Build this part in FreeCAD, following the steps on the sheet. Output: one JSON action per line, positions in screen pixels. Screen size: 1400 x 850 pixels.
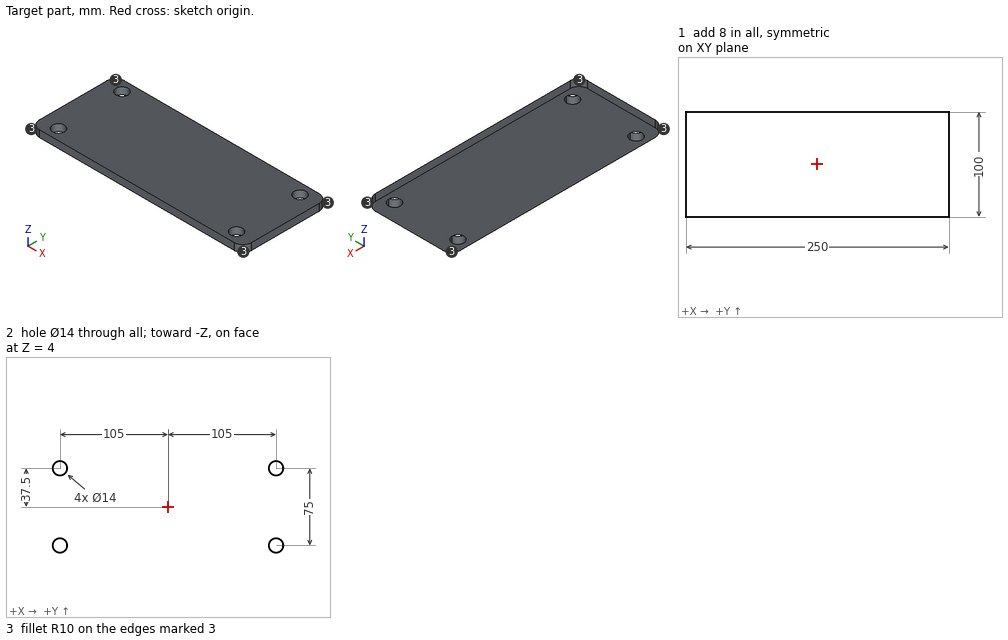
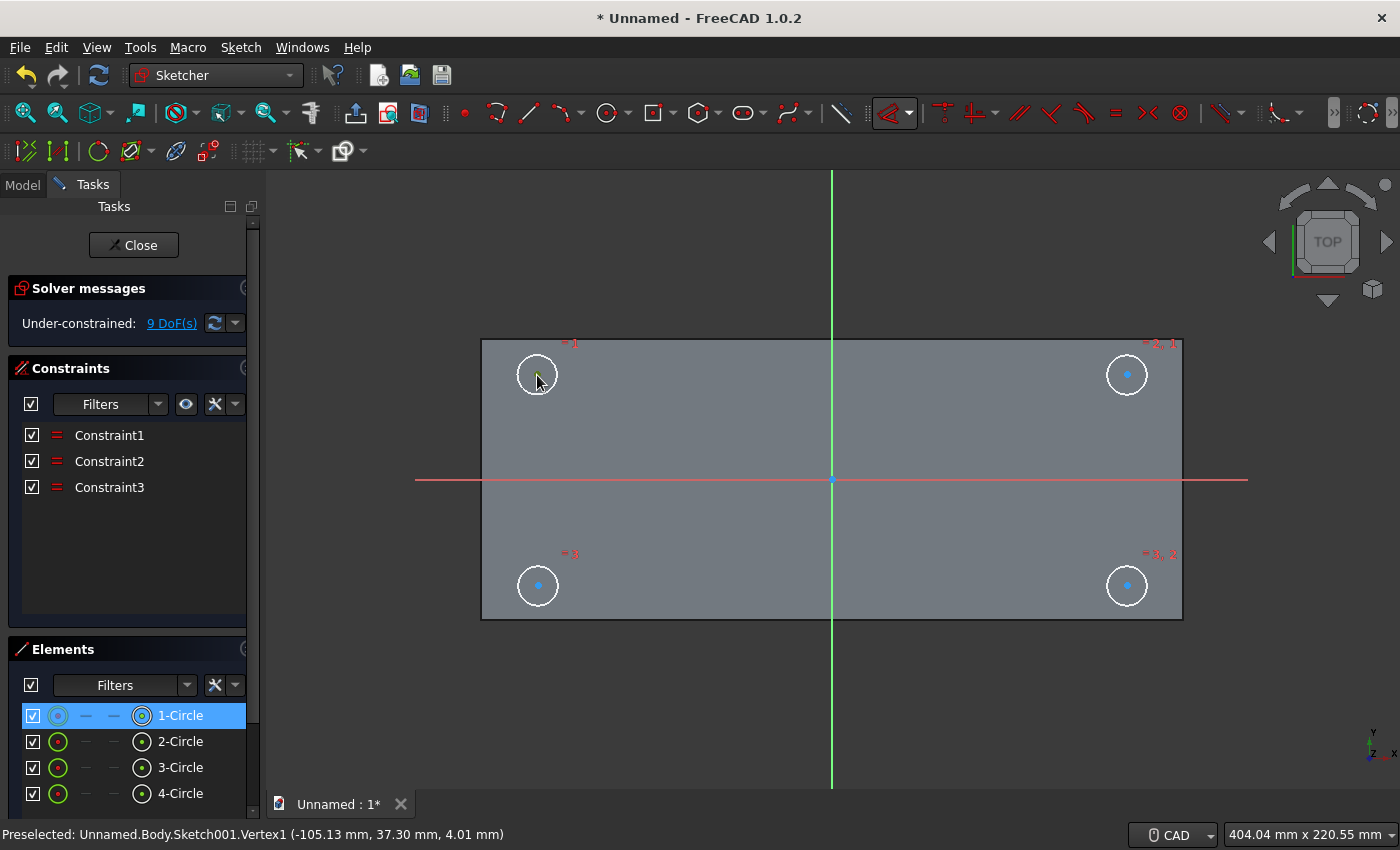
{"action": "left_click", "coordinate": [1127, 375]}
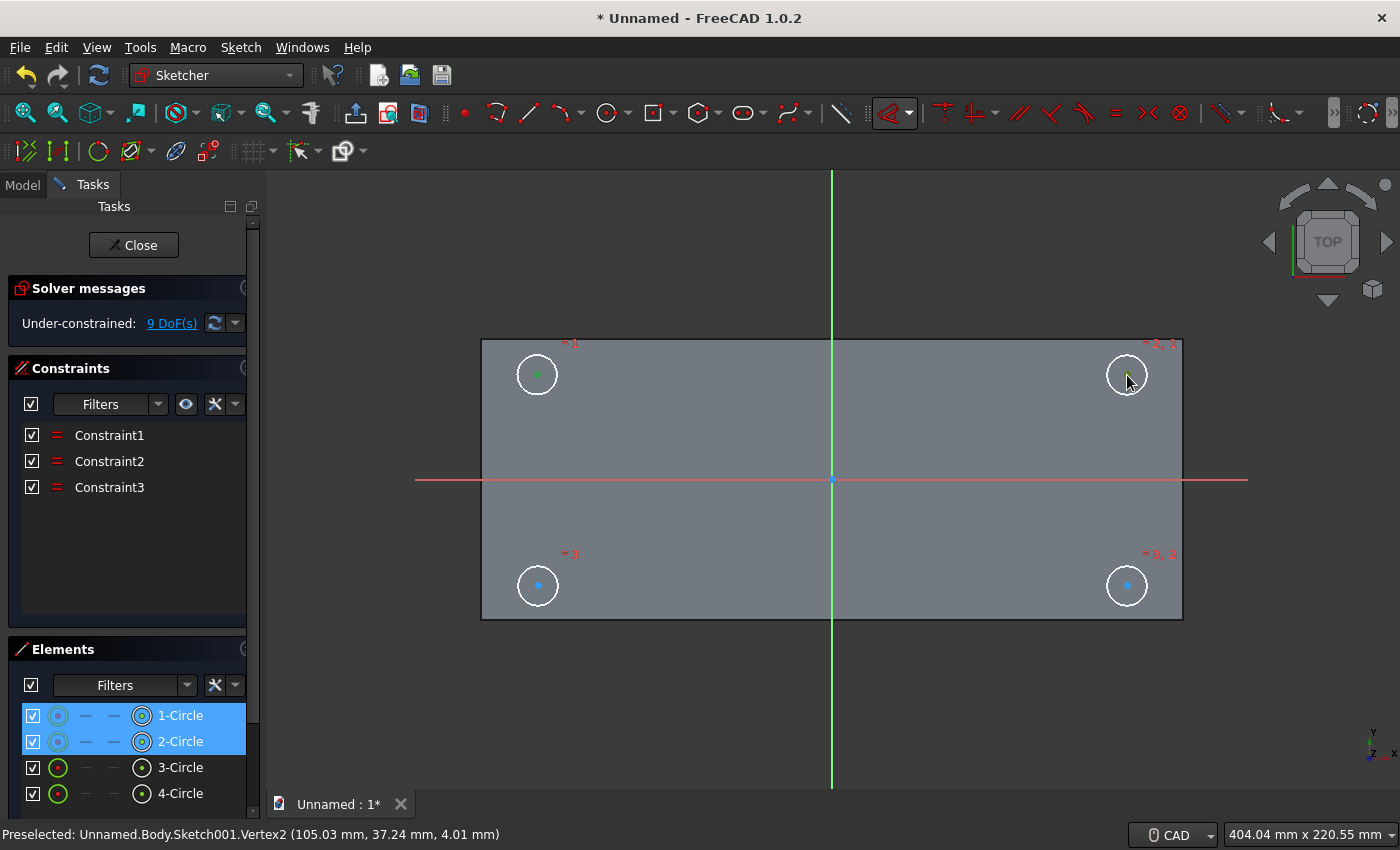
{"action": "key", "text": "h"}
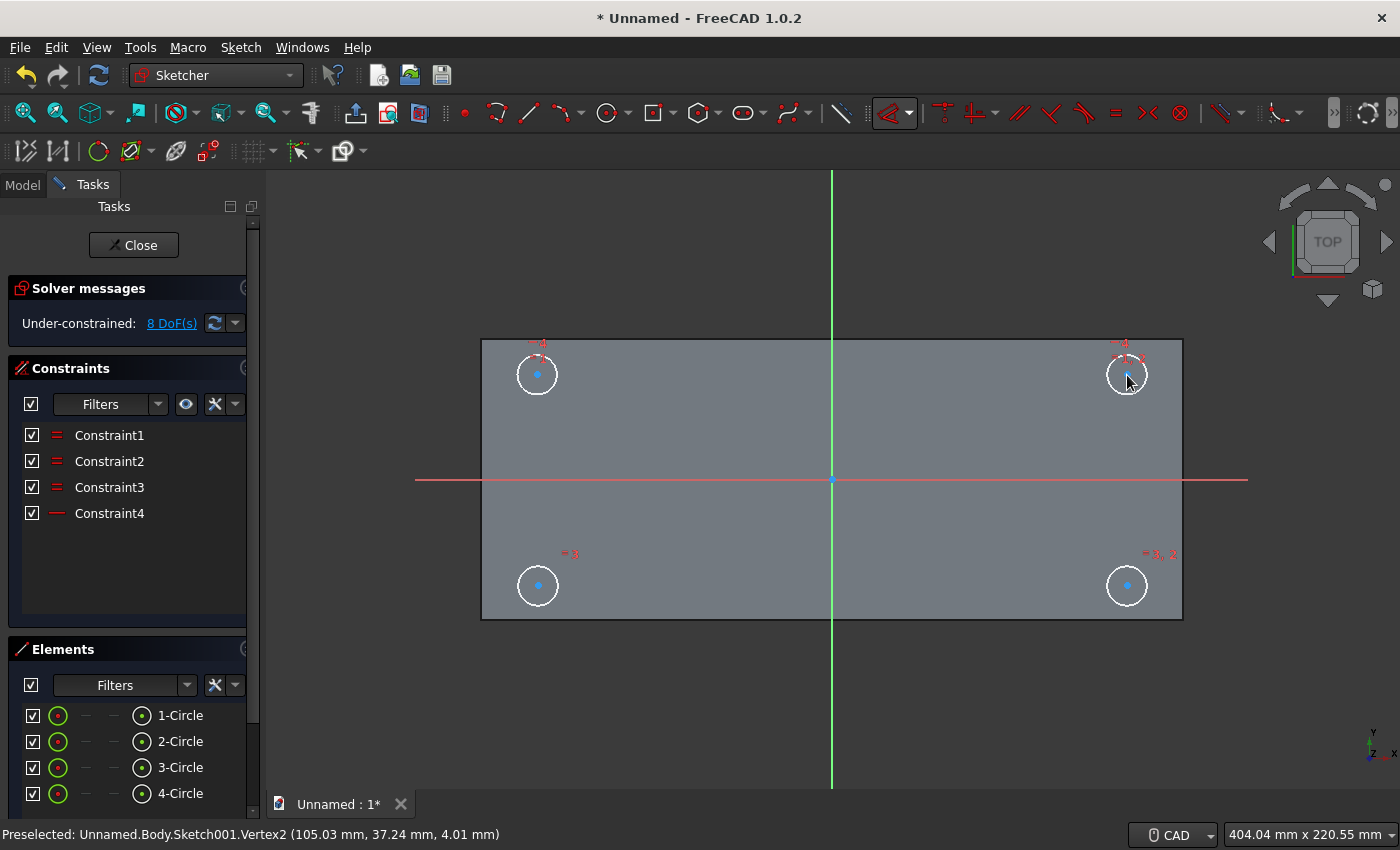
{"action": "left_click", "coordinate": [1127, 375]}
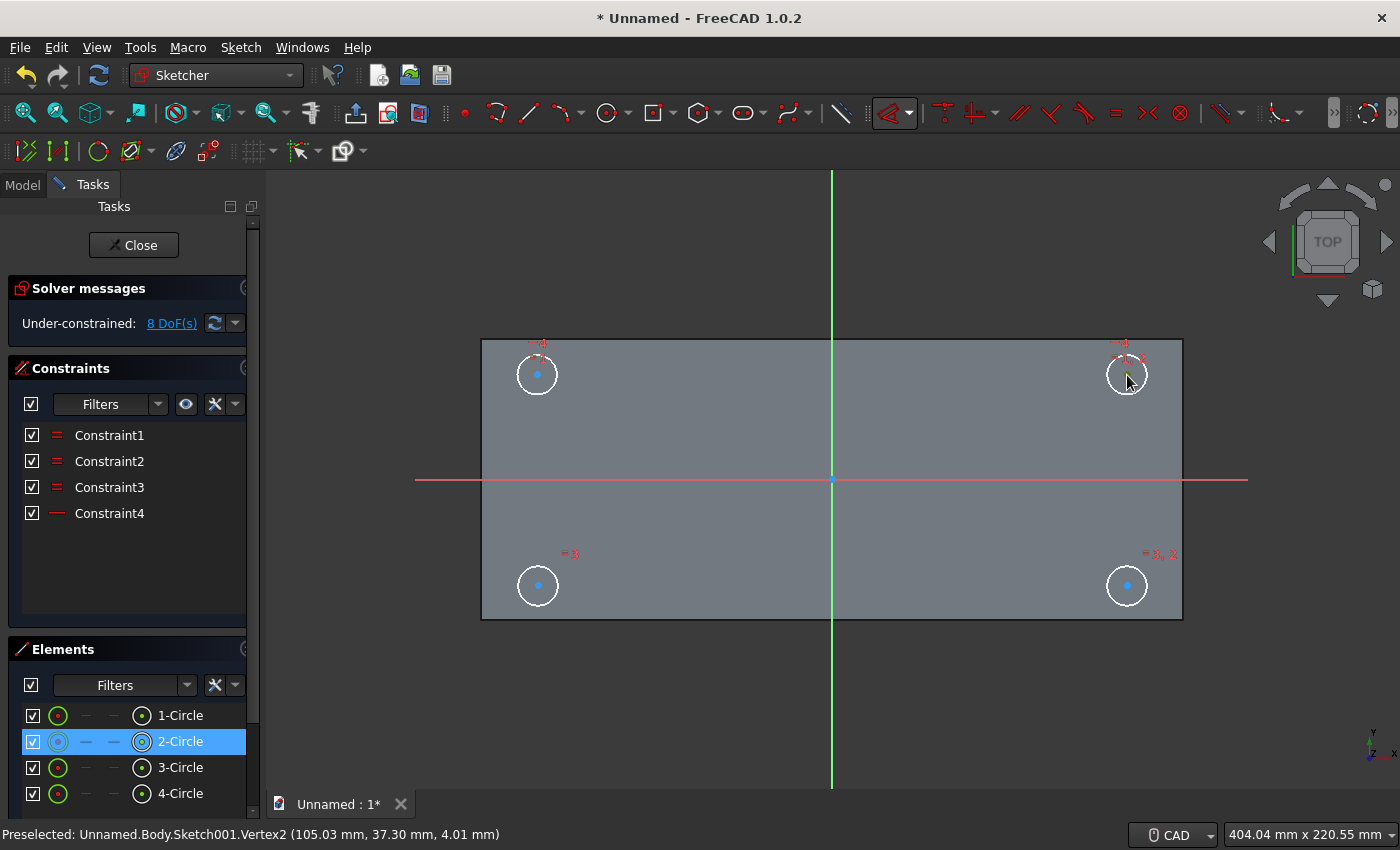
{"action": "left_click", "coordinate": [1127, 586]}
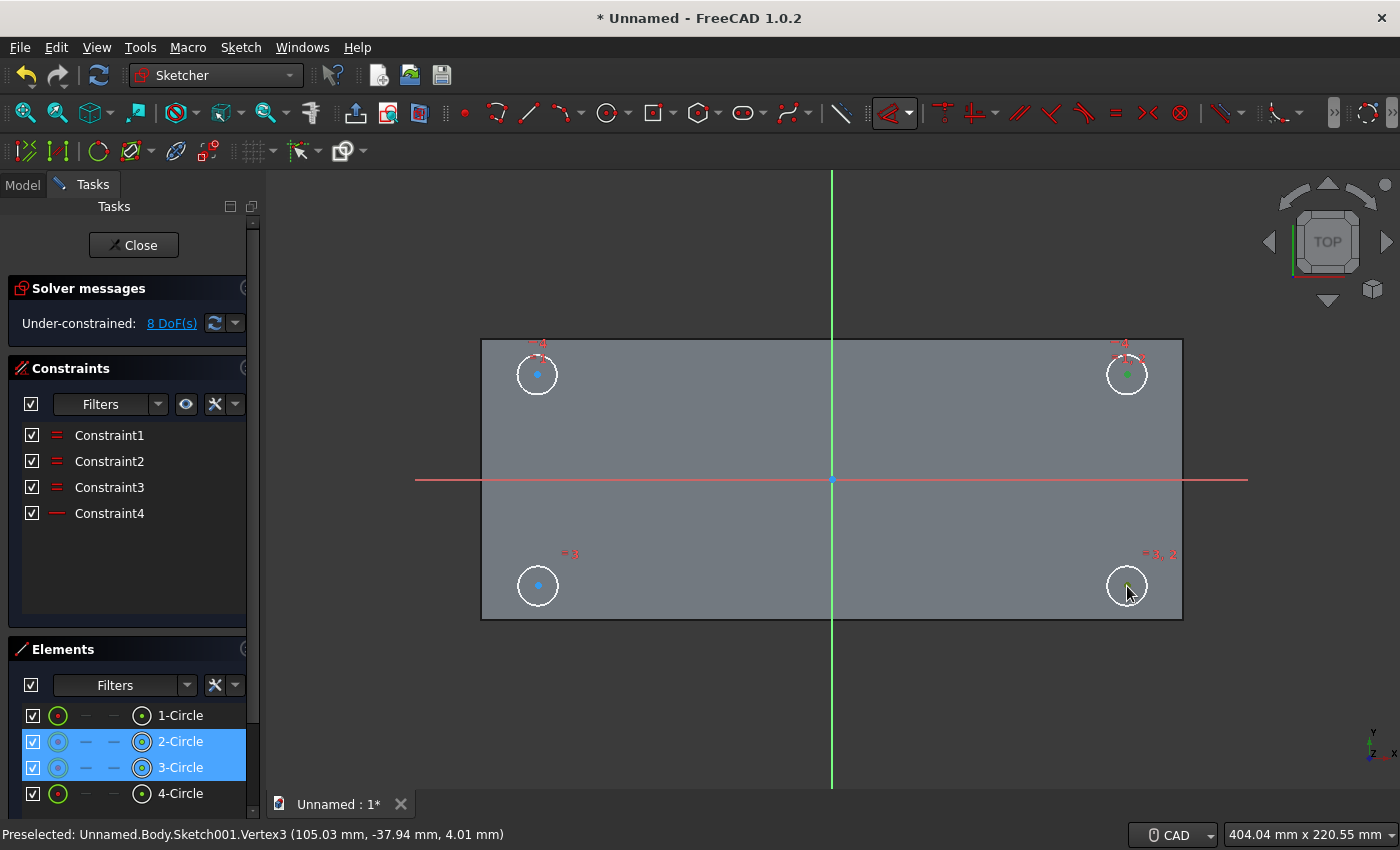
{"action": "left_click", "coordinate": [998, 114]}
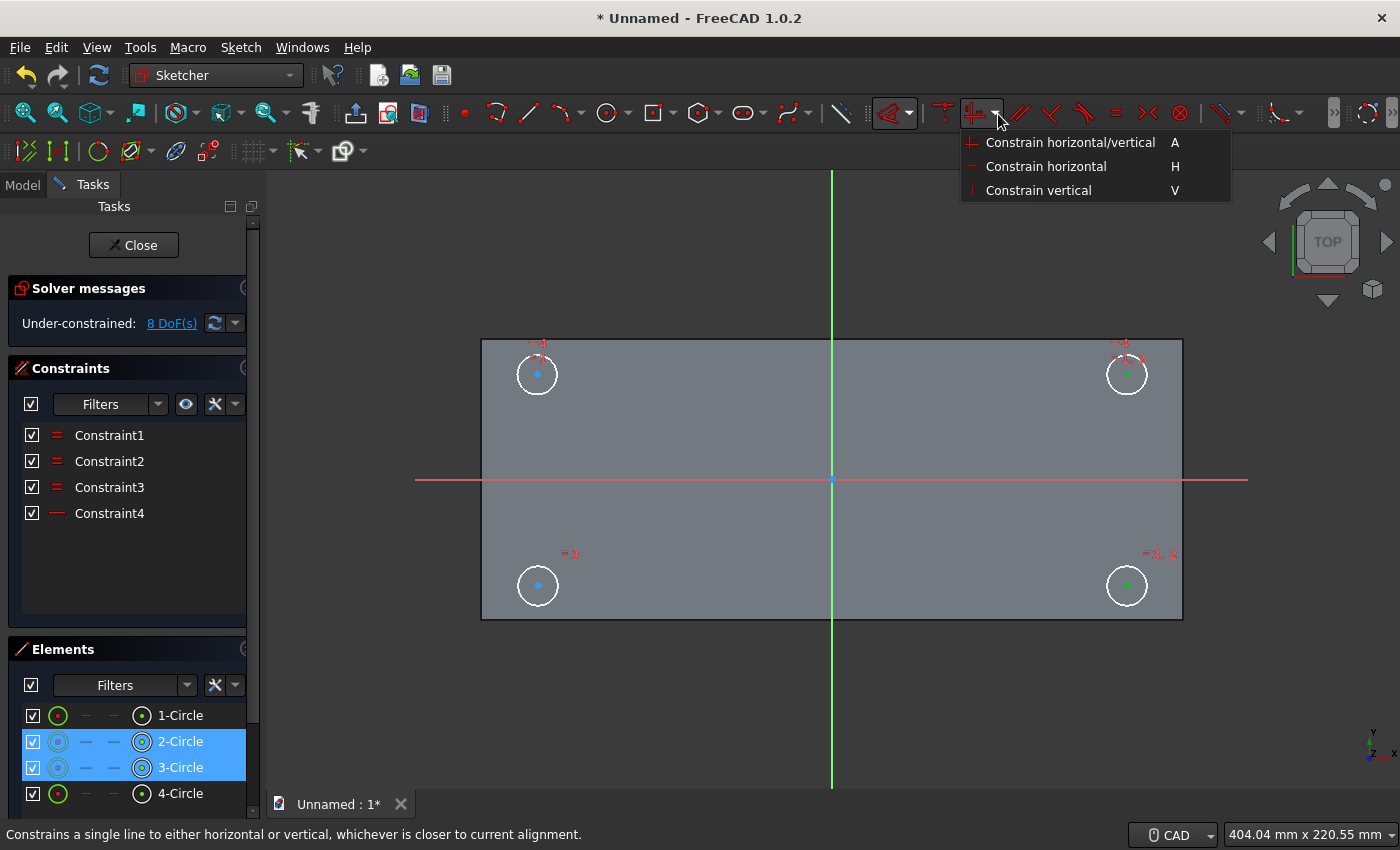
{"action": "left_click", "coordinate": [1096, 190]}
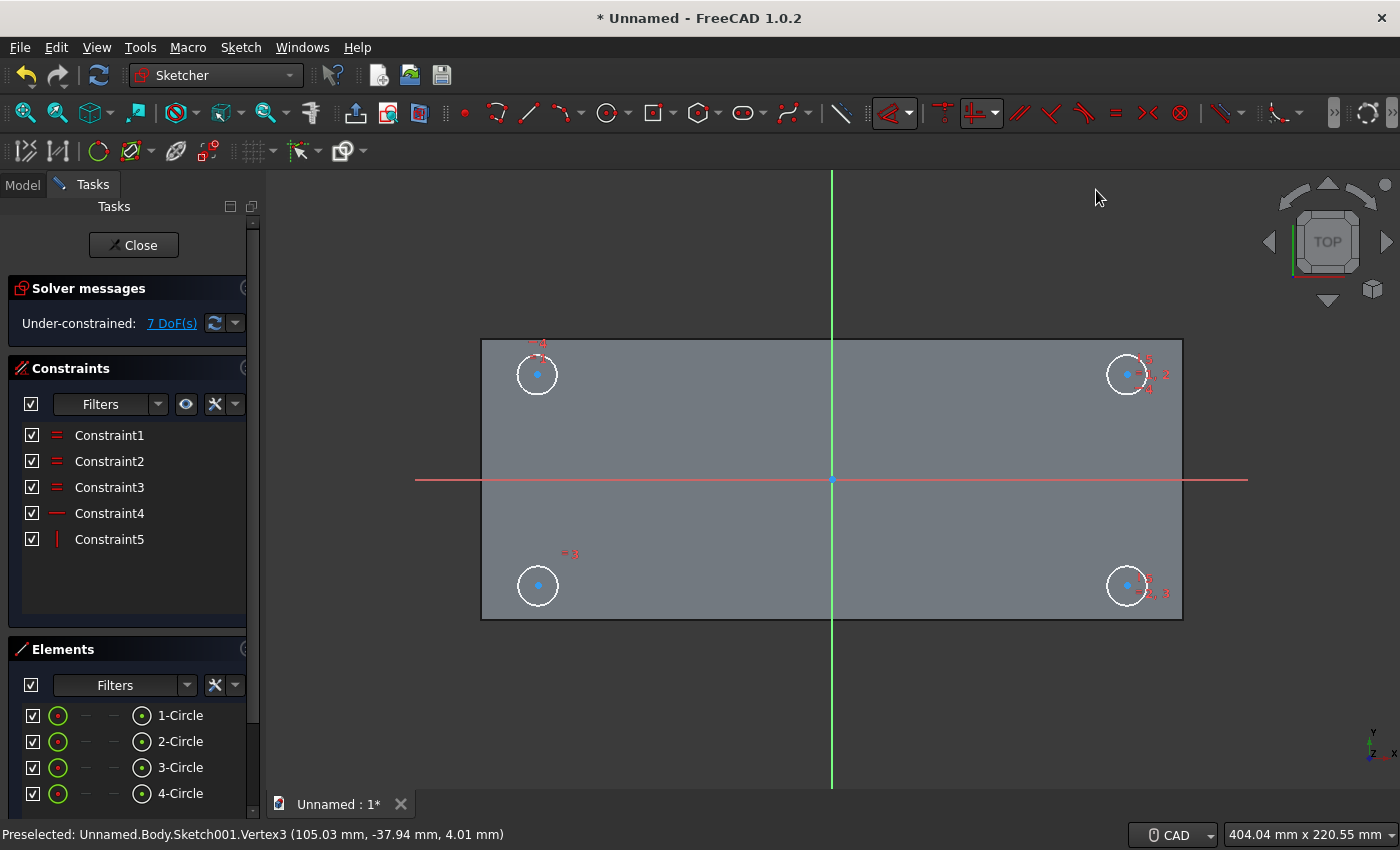
{"action": "left_click", "coordinate": [537, 375]}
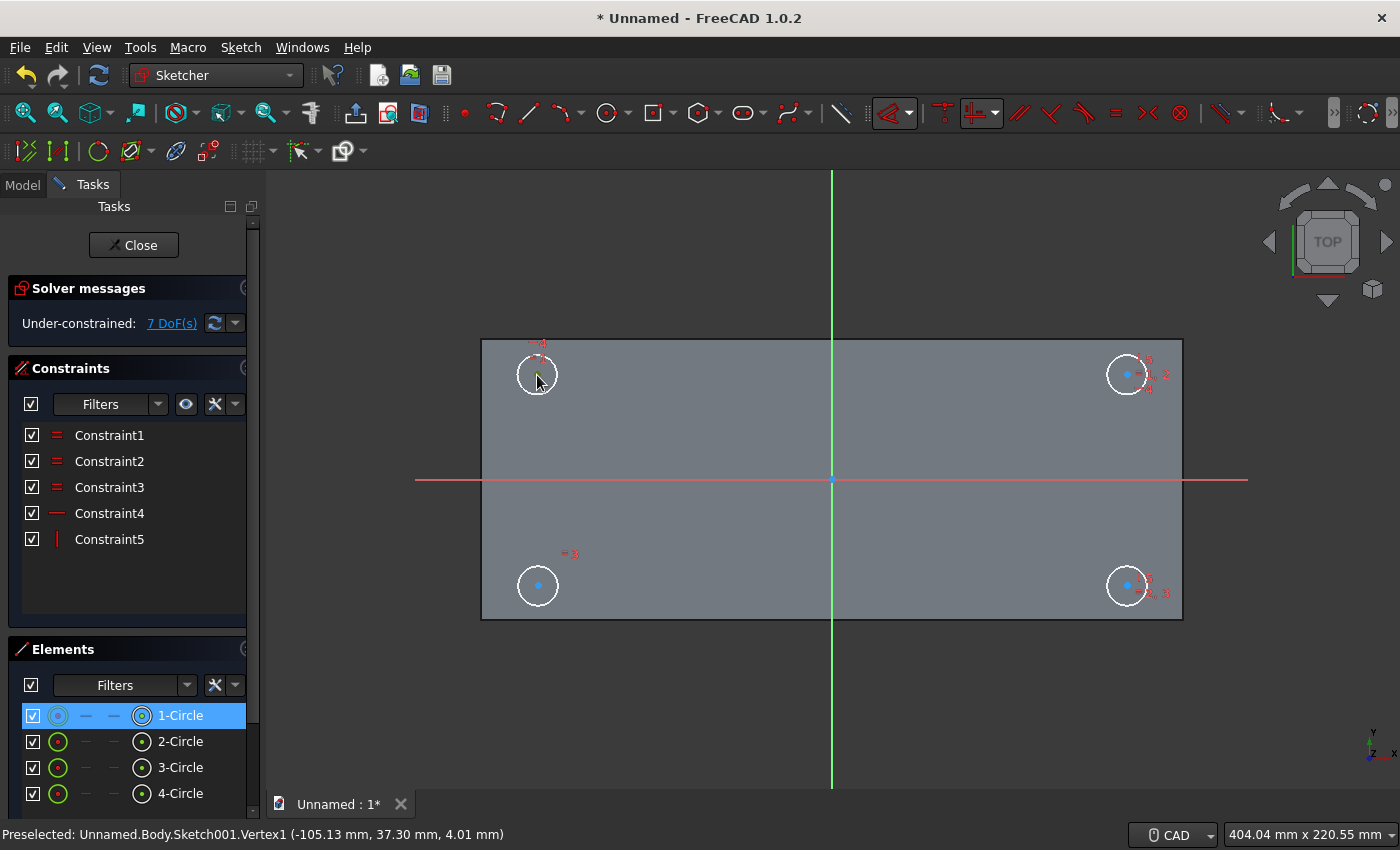
{"action": "left_click", "coordinate": [538, 586]}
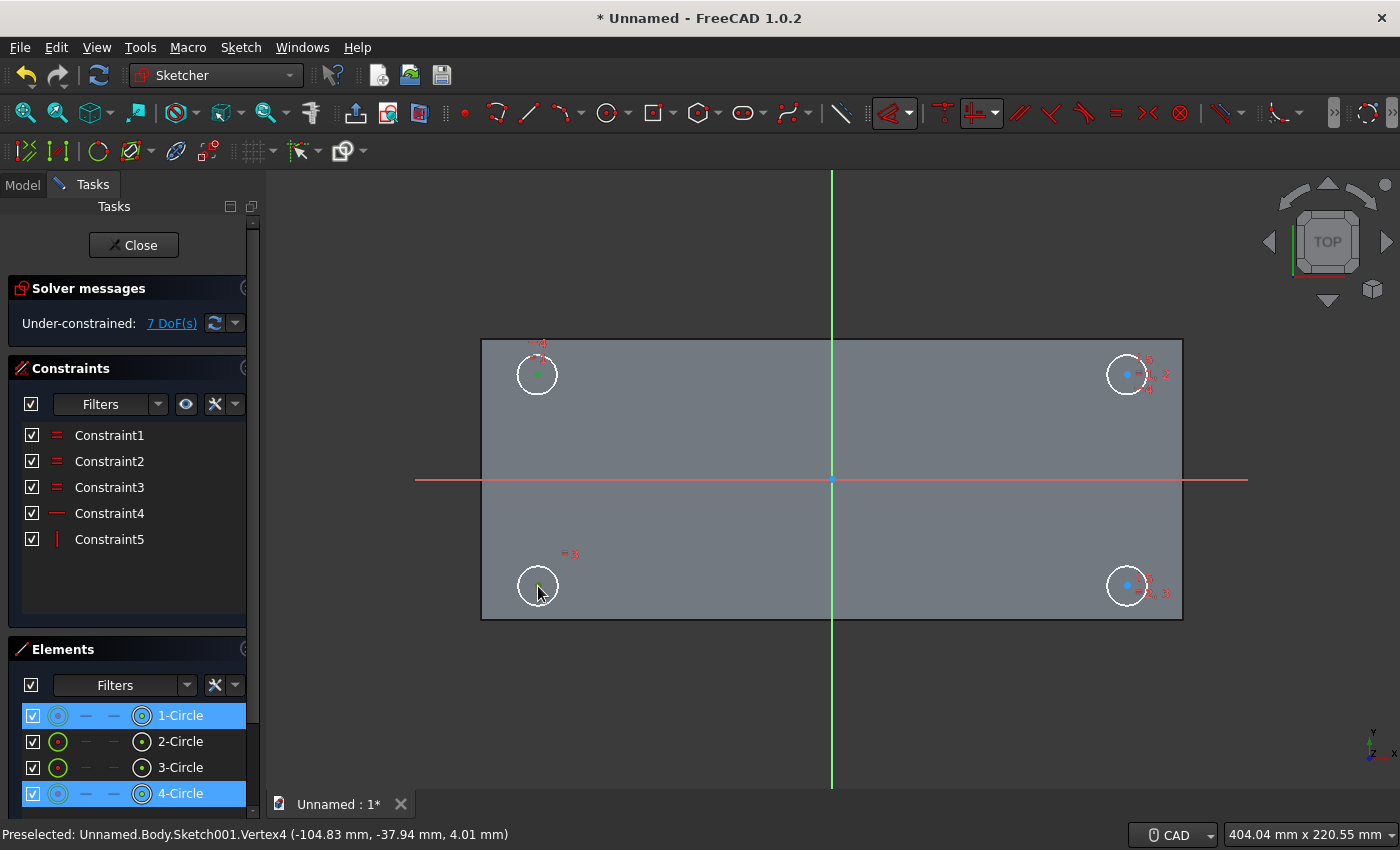
{"action": "left_click", "coordinate": [998, 114]}